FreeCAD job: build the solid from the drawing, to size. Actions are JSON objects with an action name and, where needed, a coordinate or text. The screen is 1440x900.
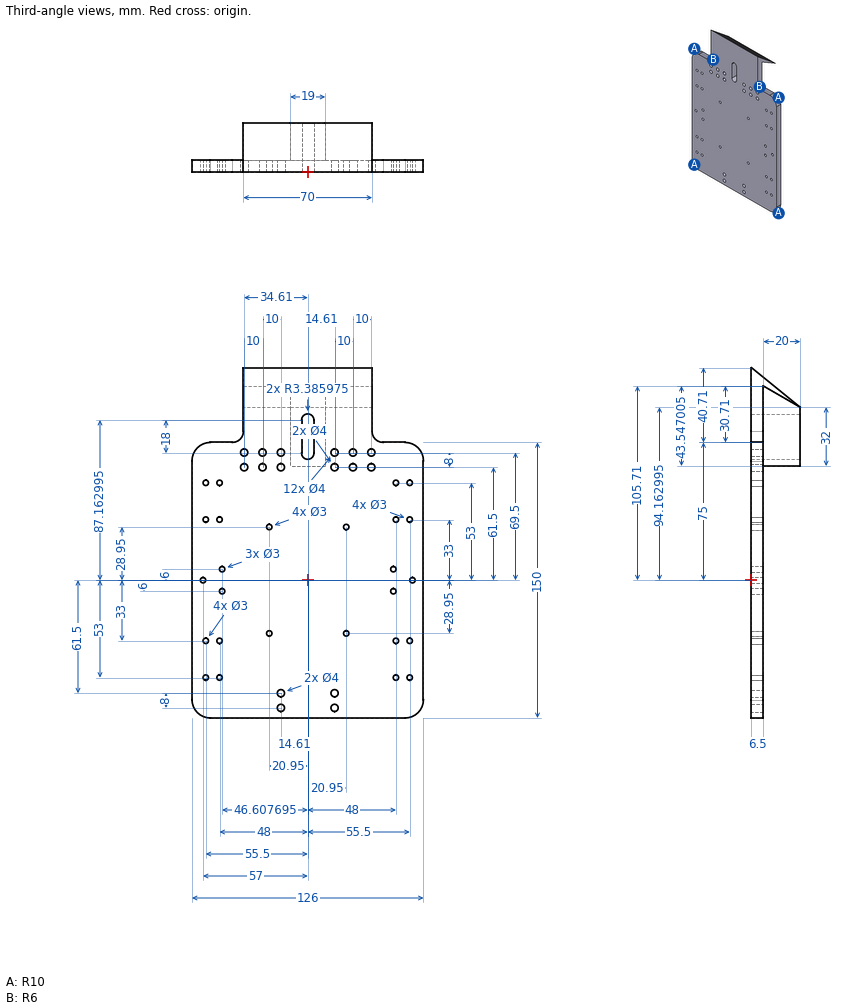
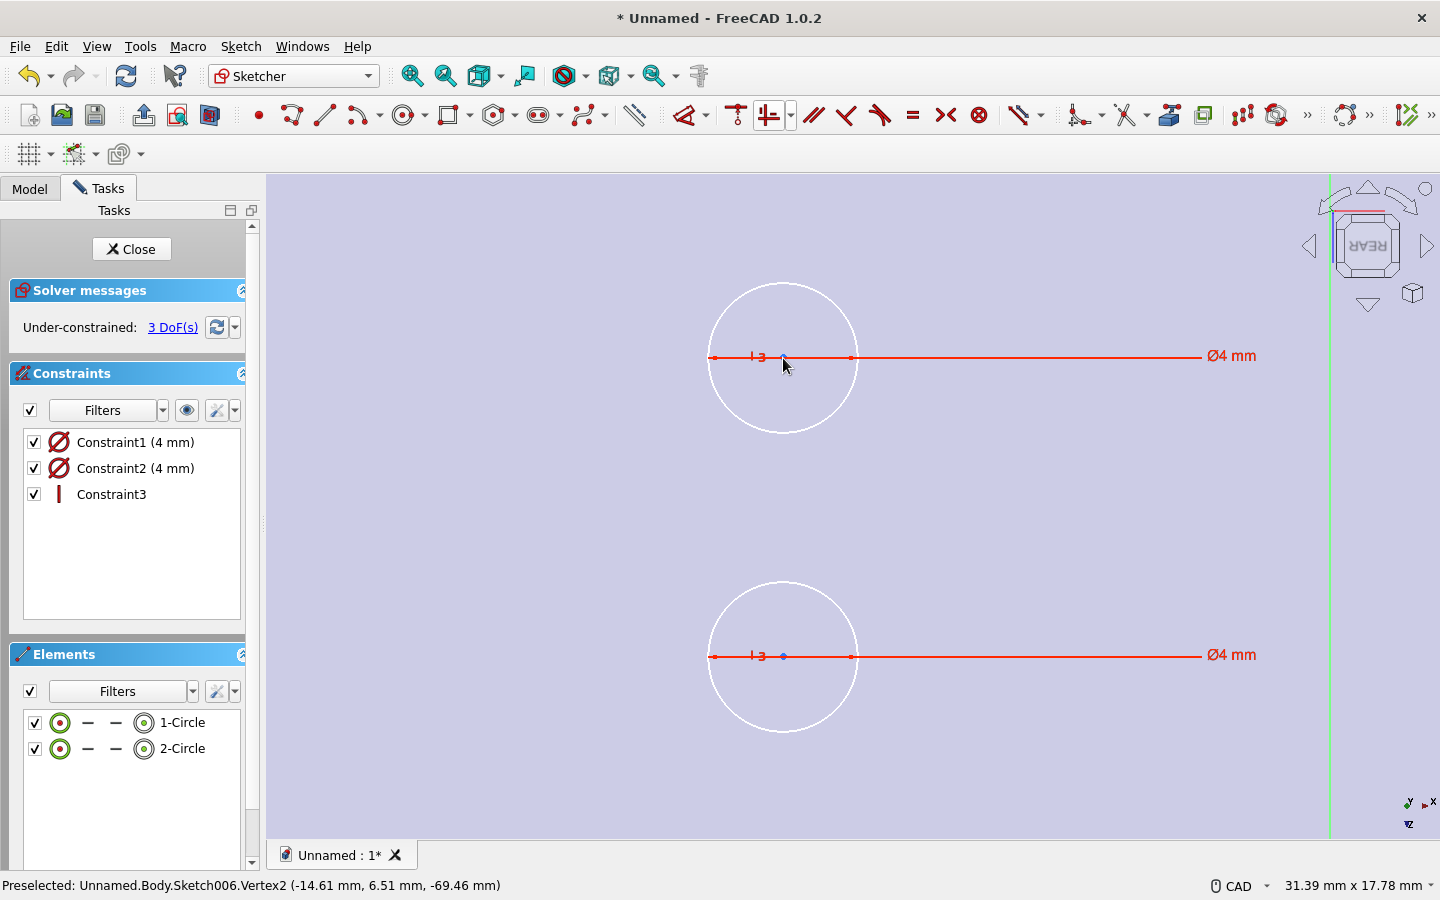
{"action": "left_click", "coordinate": [684, 116]}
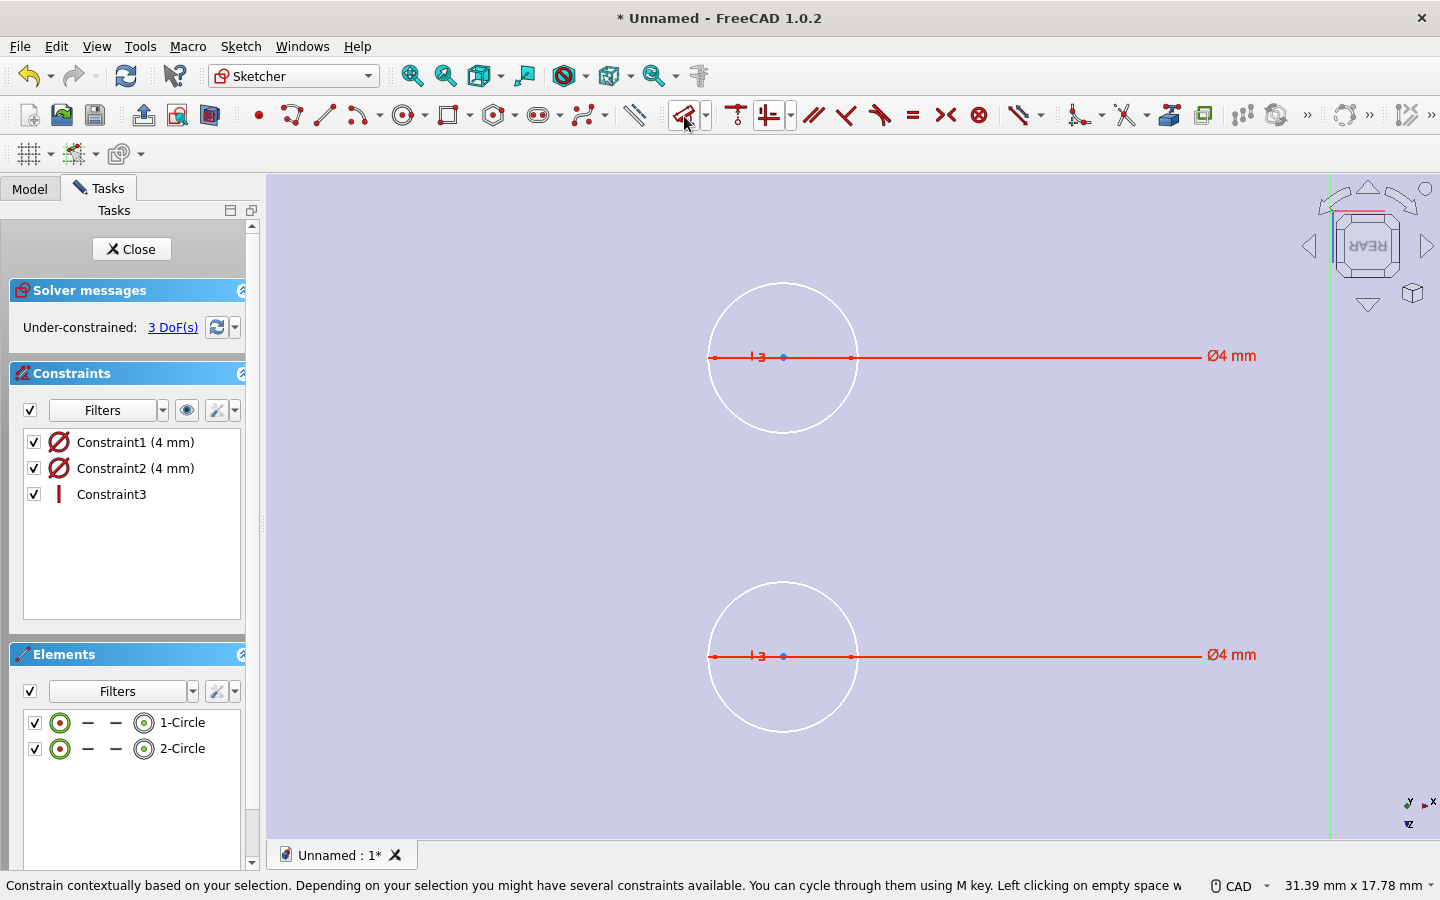
{"action": "left_click", "coordinate": [783, 657]}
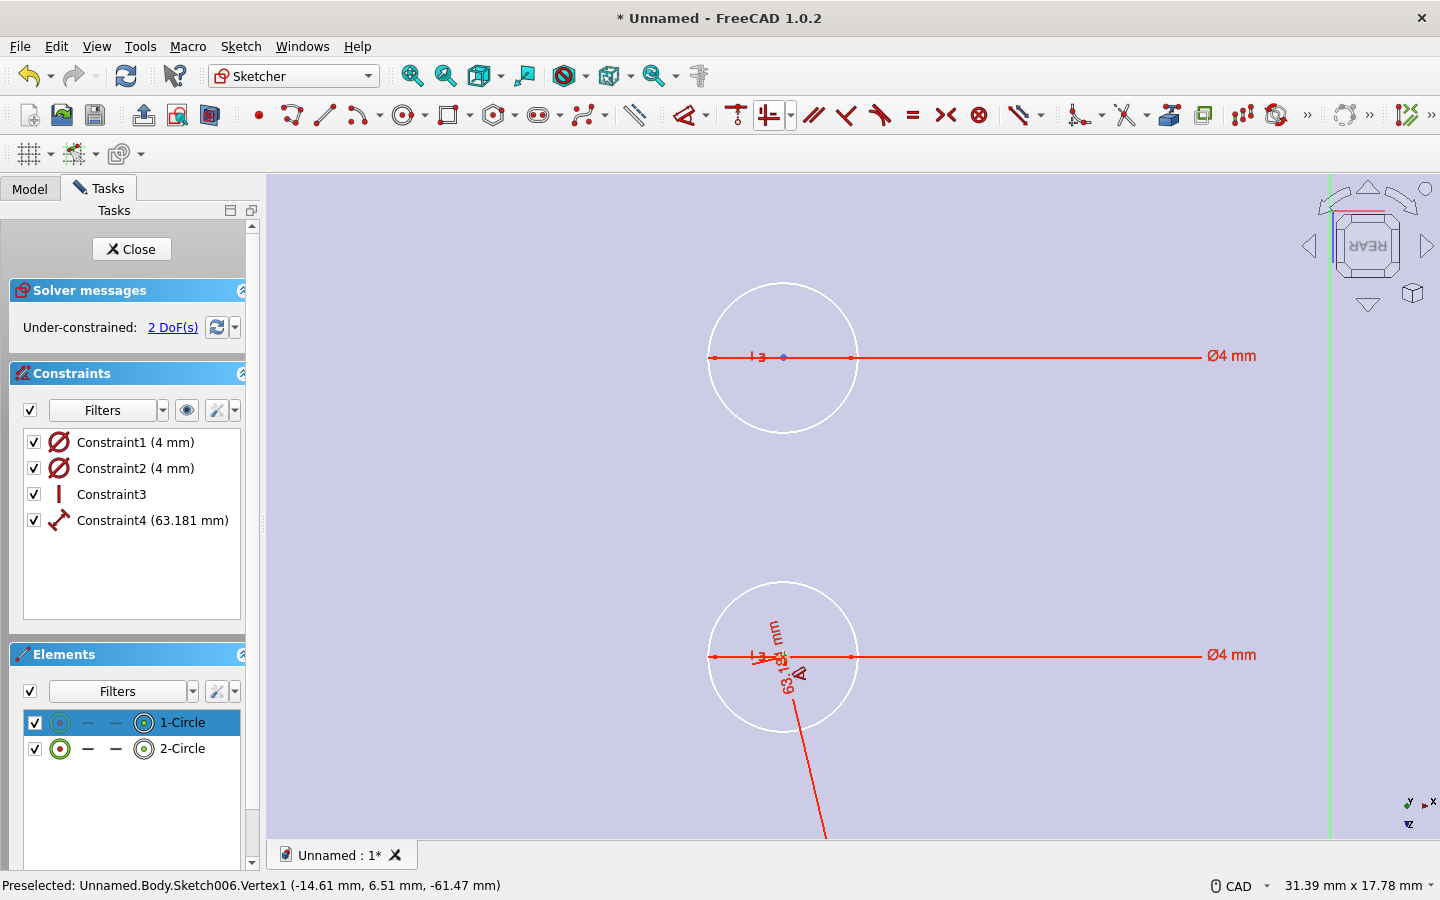
{"action": "left_click", "coordinate": [783, 358]}
{"action": "left_click", "coordinate": [749, 508]}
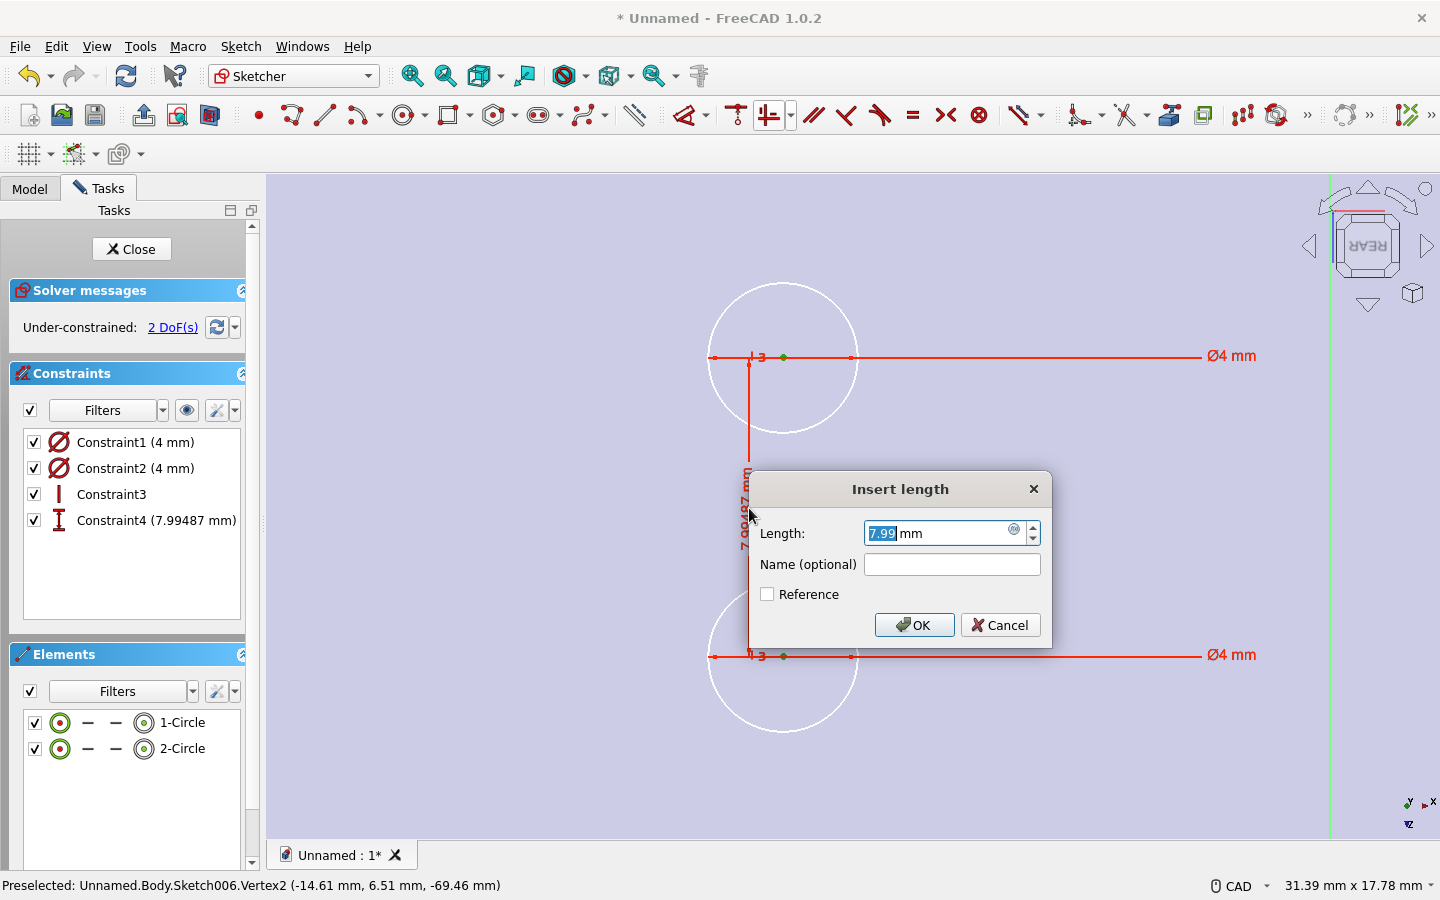
{"action": "type", "text": "8"}
{"action": "key", "text": "Return"}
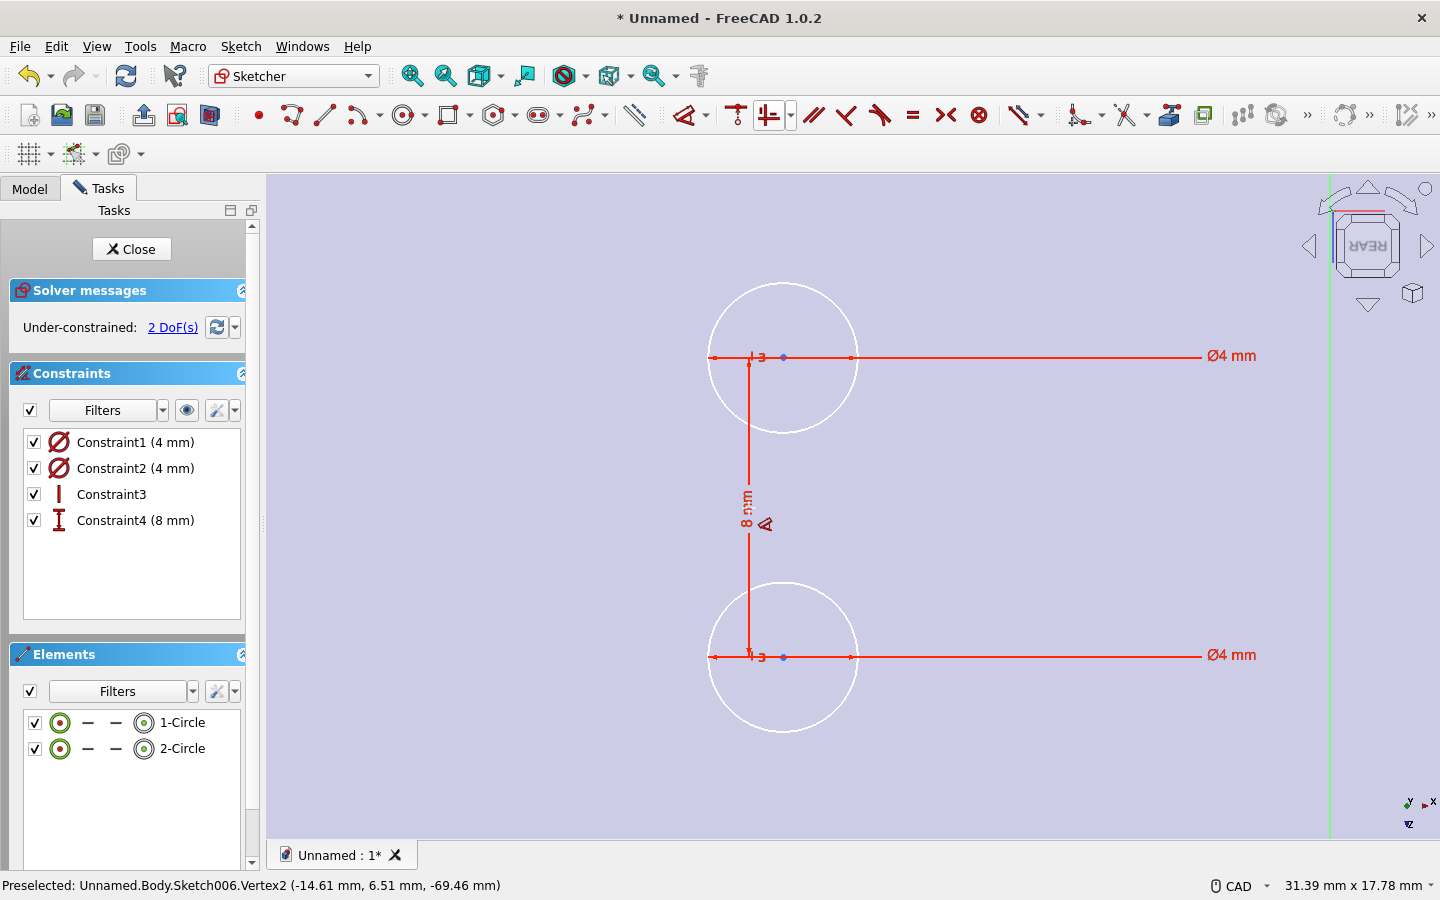
{"action": "left_click", "coordinate": [783, 657]}
{"action": "left_click", "coordinate": [749, 699]}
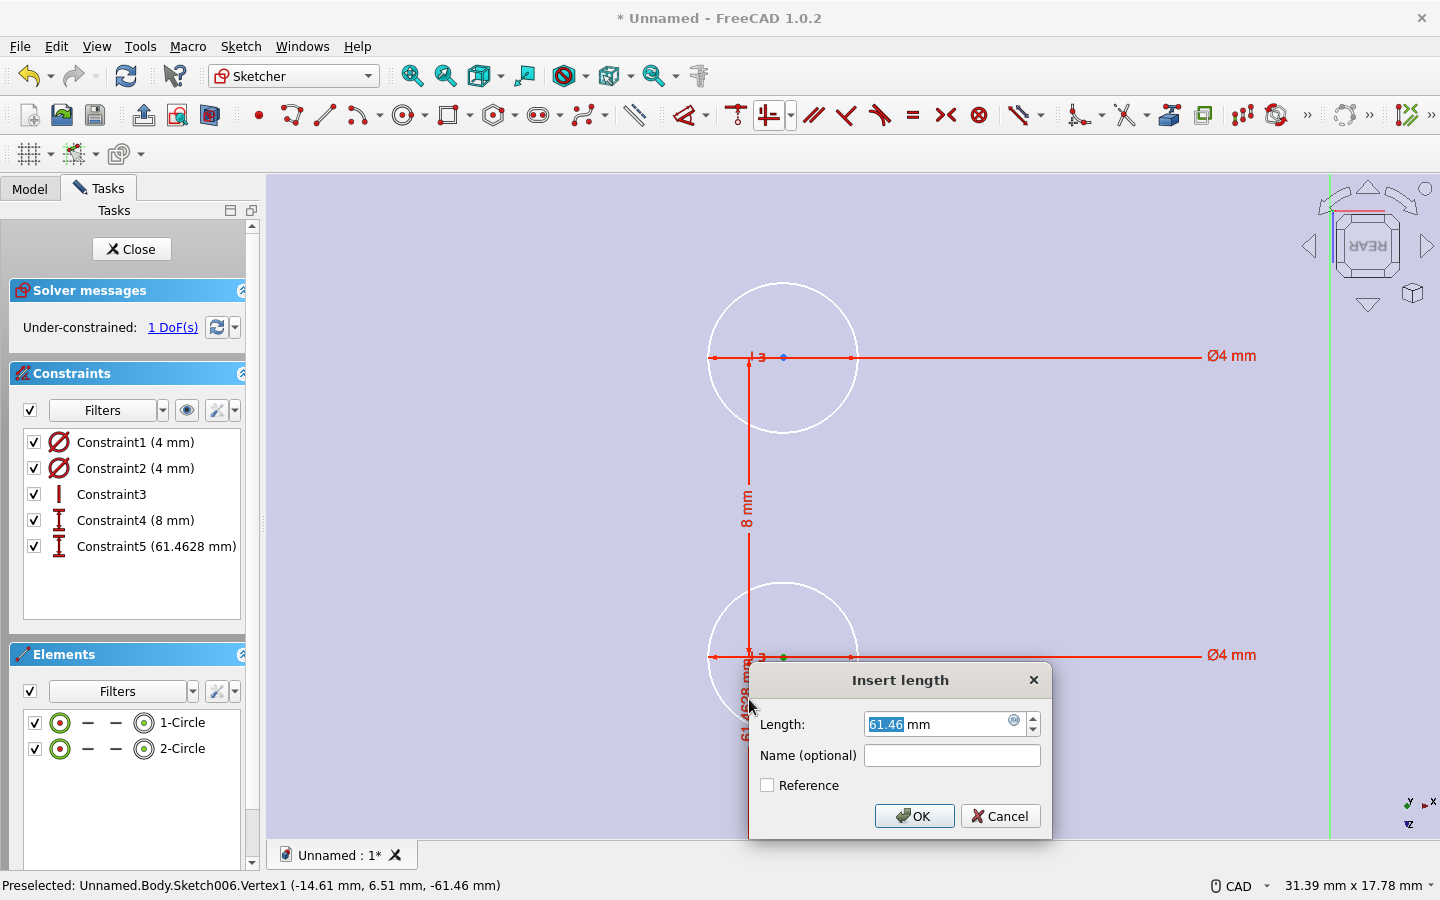
{"action": "type", "text": "61.5"}
{"action": "key", "text": "Return"}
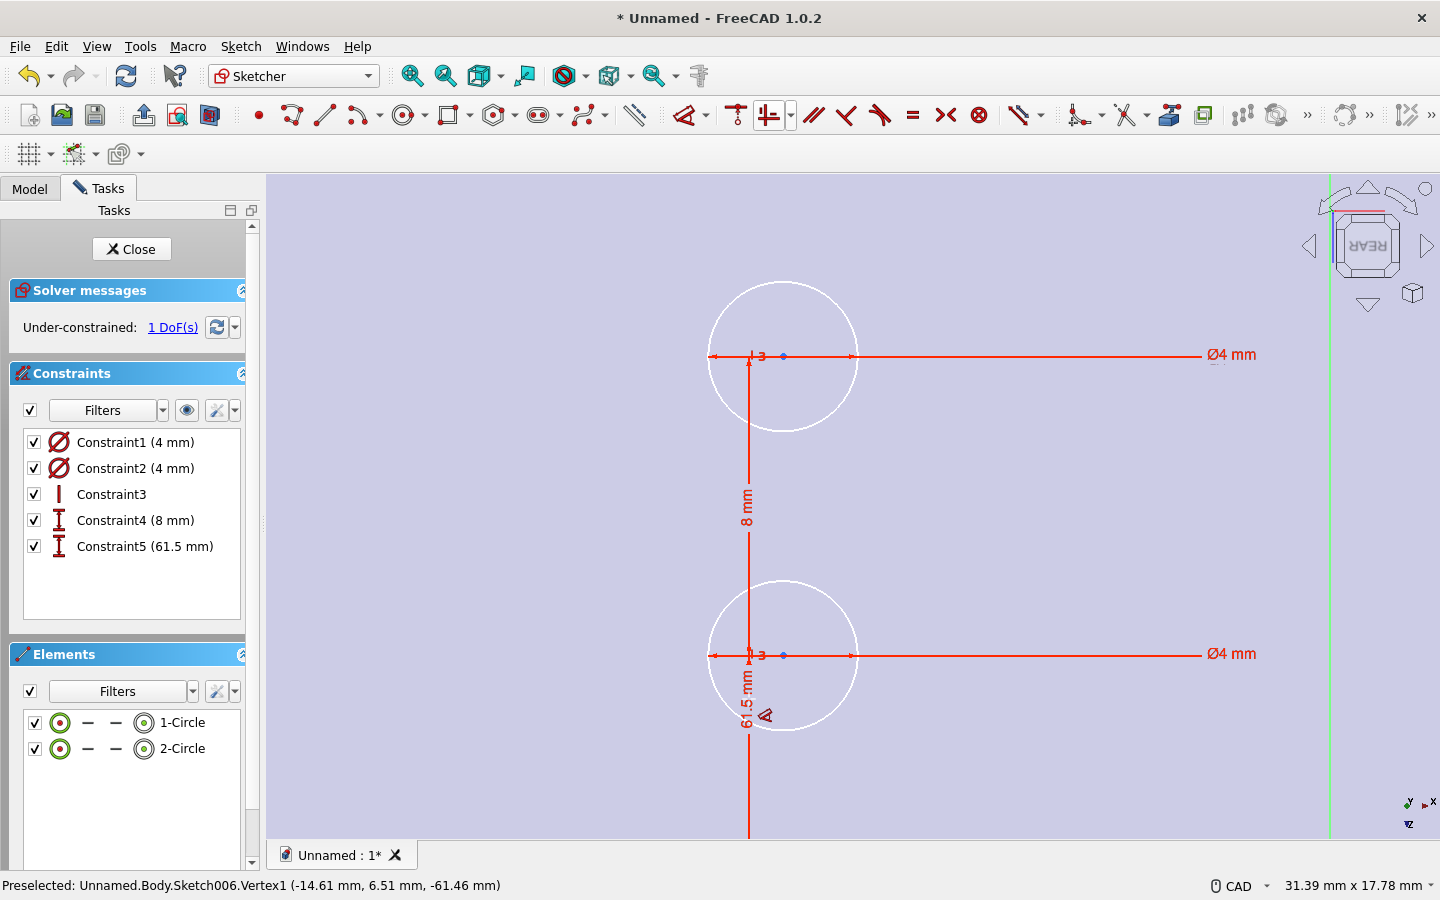
{"action": "left_click", "coordinate": [783, 656]}
{"action": "left_click", "coordinate": [1029, 622]}